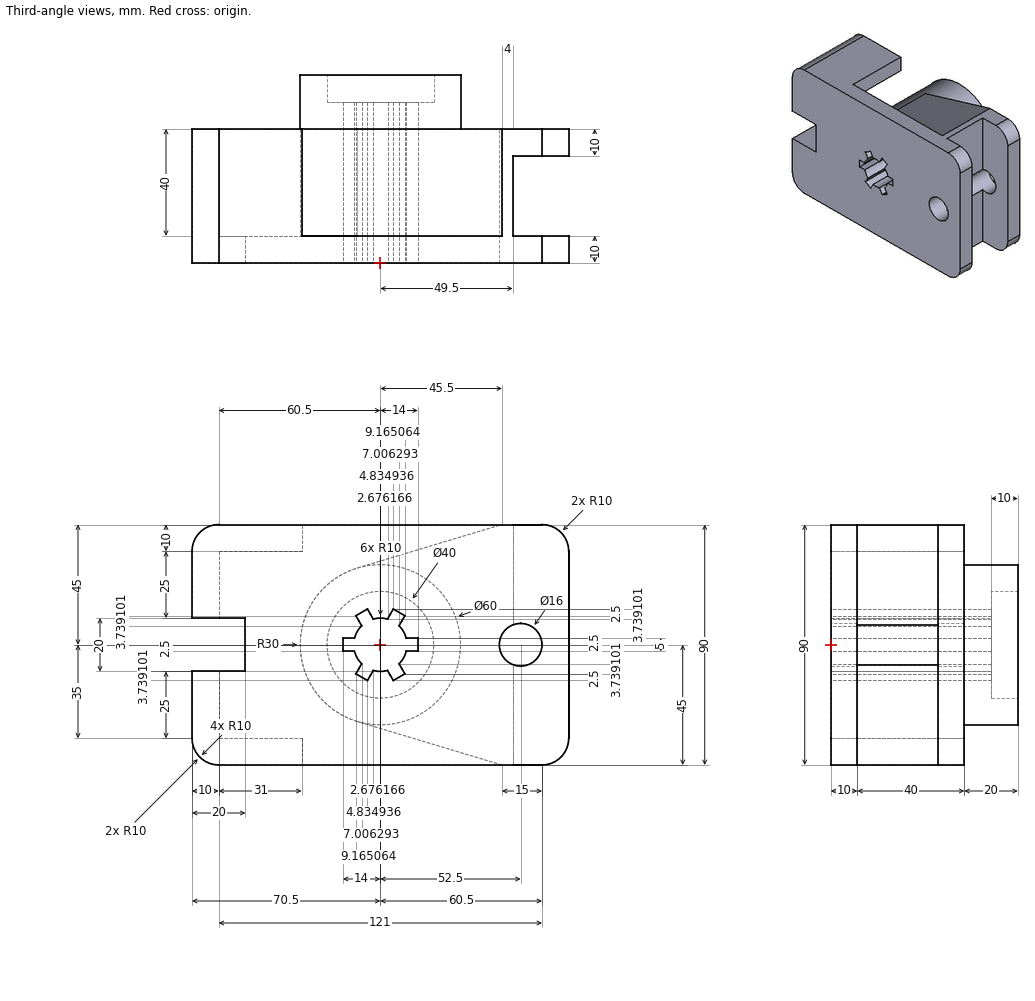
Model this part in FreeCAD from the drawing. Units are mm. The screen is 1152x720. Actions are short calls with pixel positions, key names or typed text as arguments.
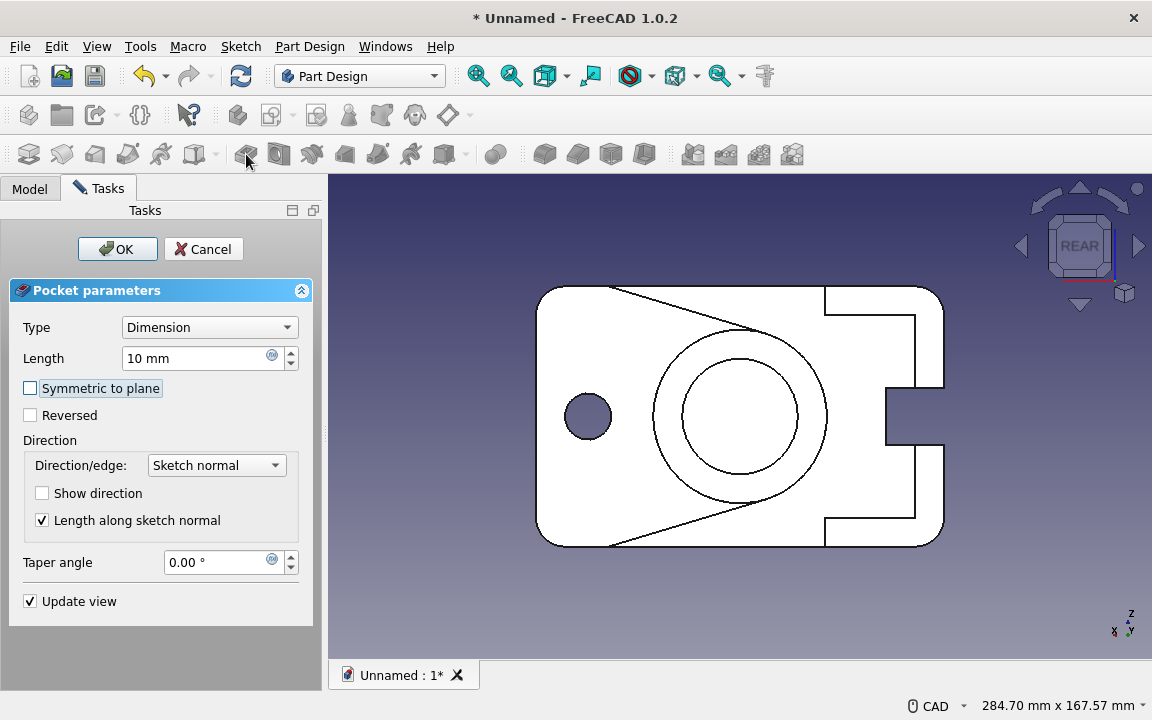
click(118, 249)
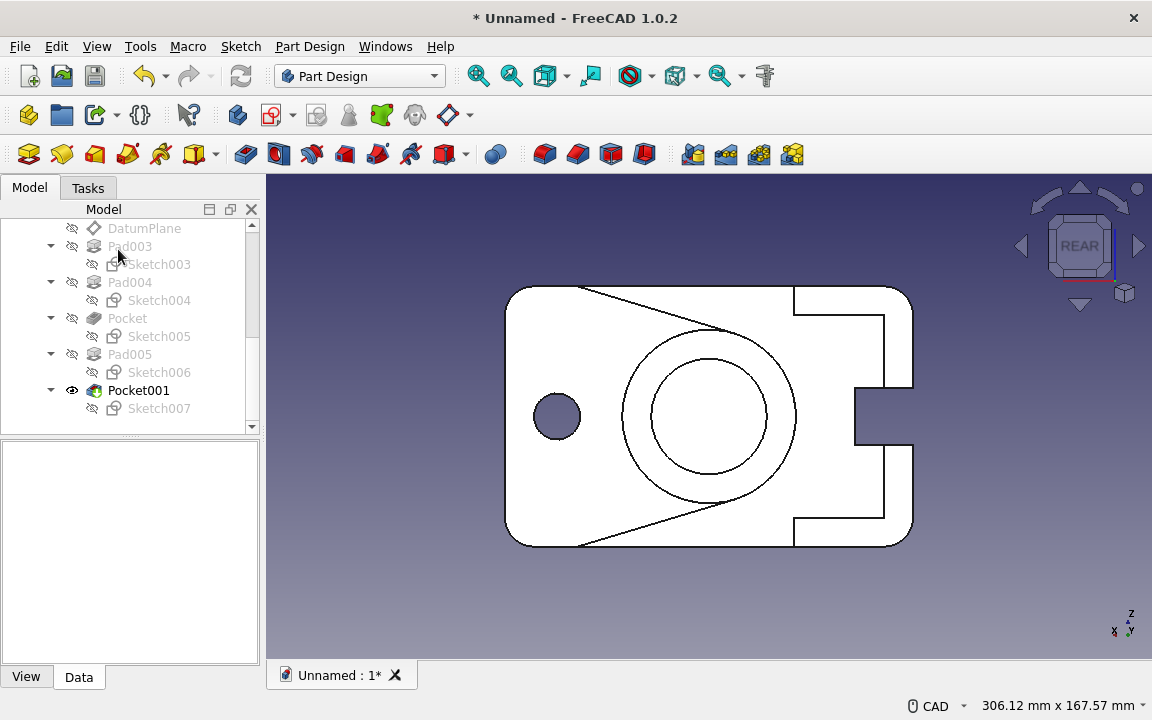
click(709, 416)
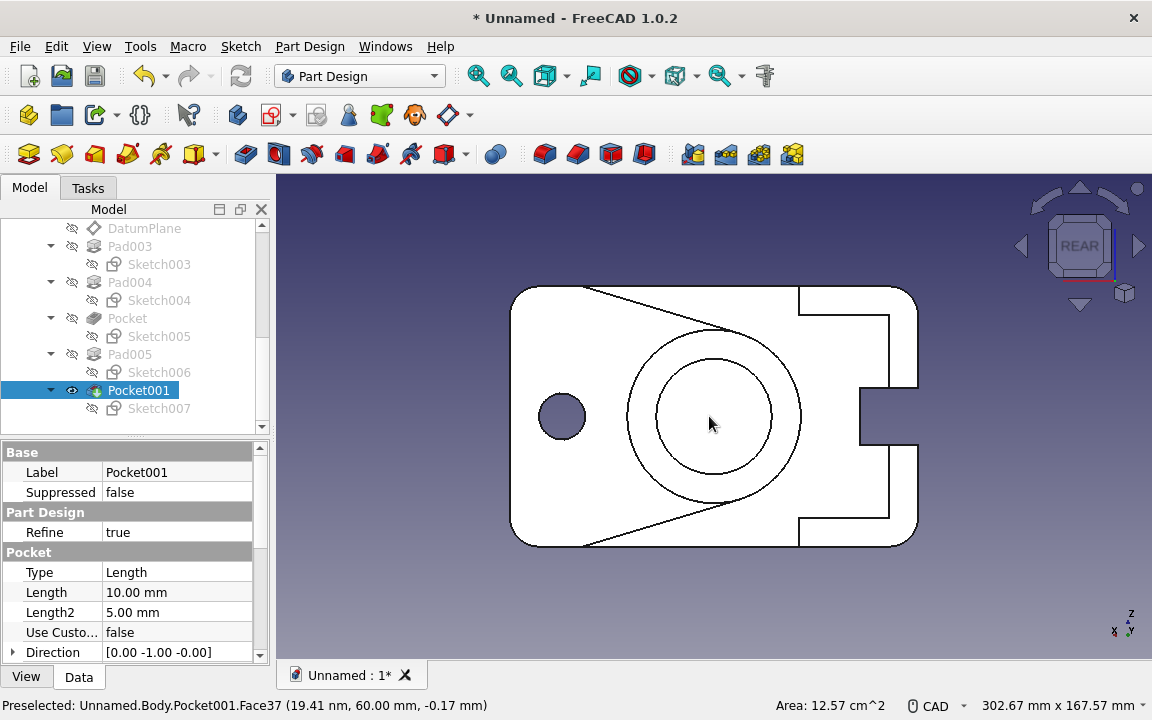
click(270, 116)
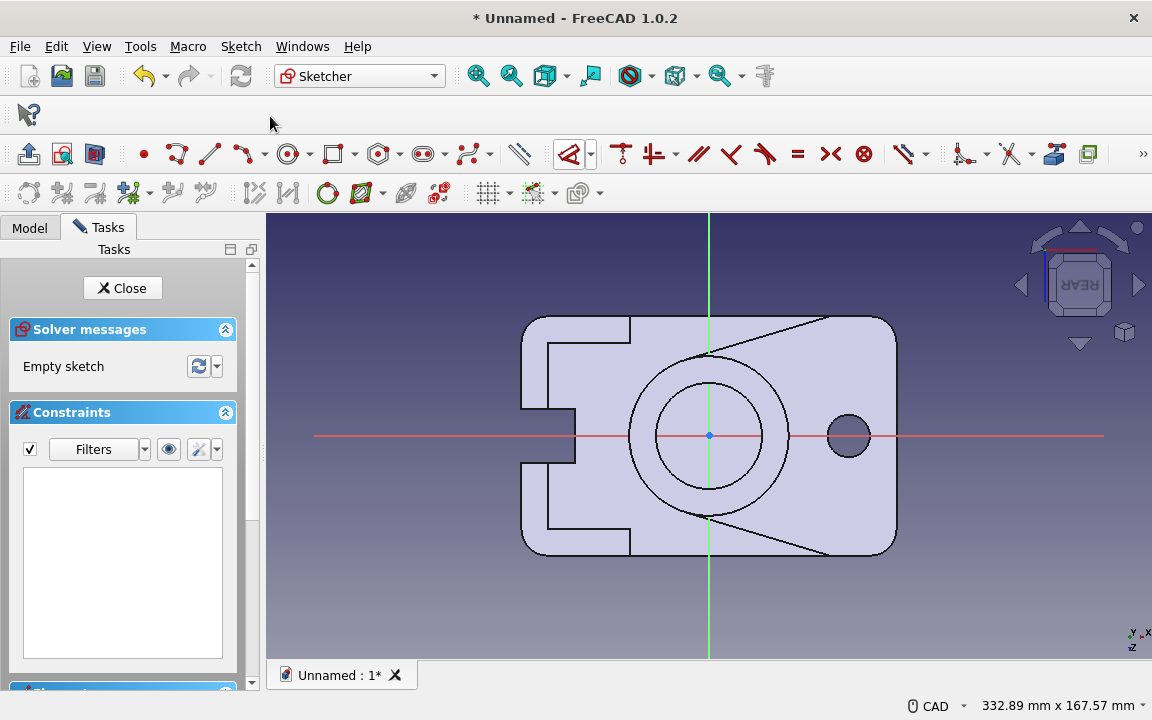
click(95, 154)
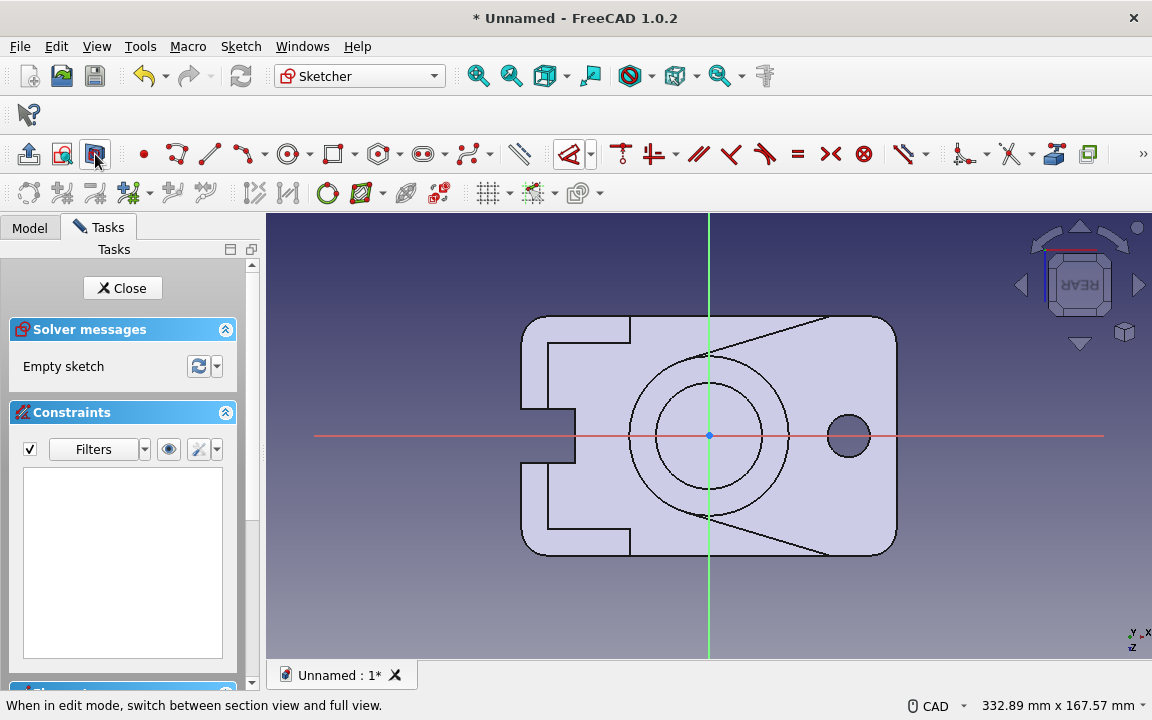
scroll(731, 436, up, 7)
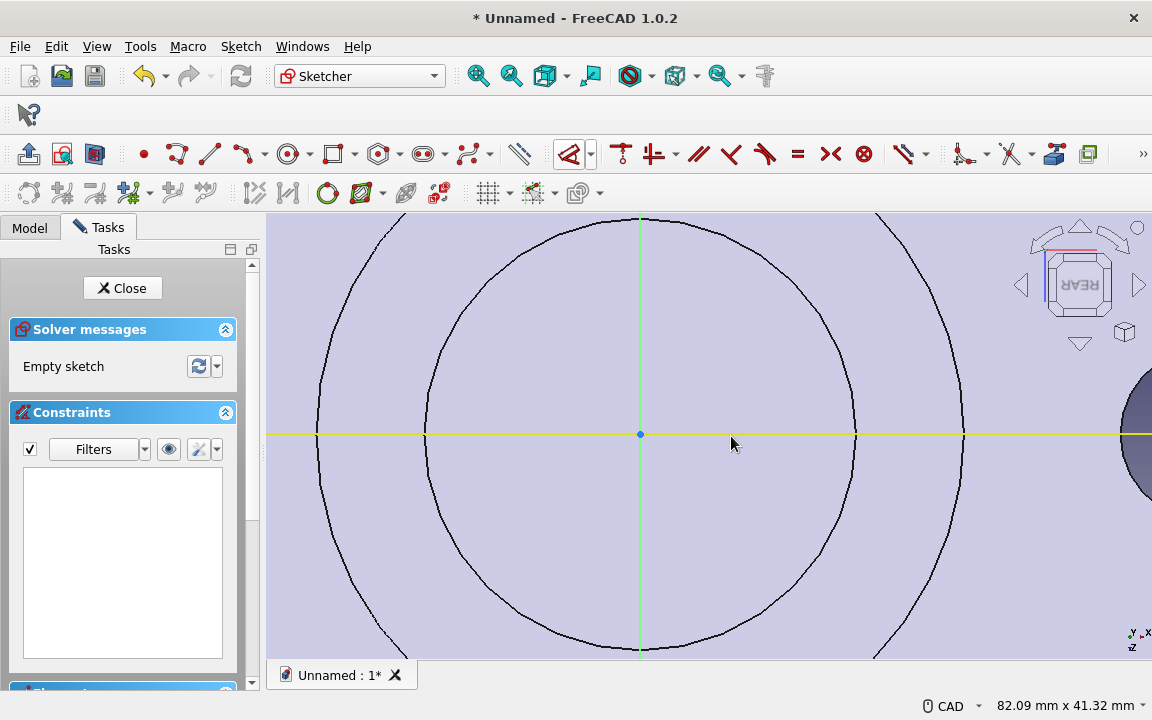
click(177, 154)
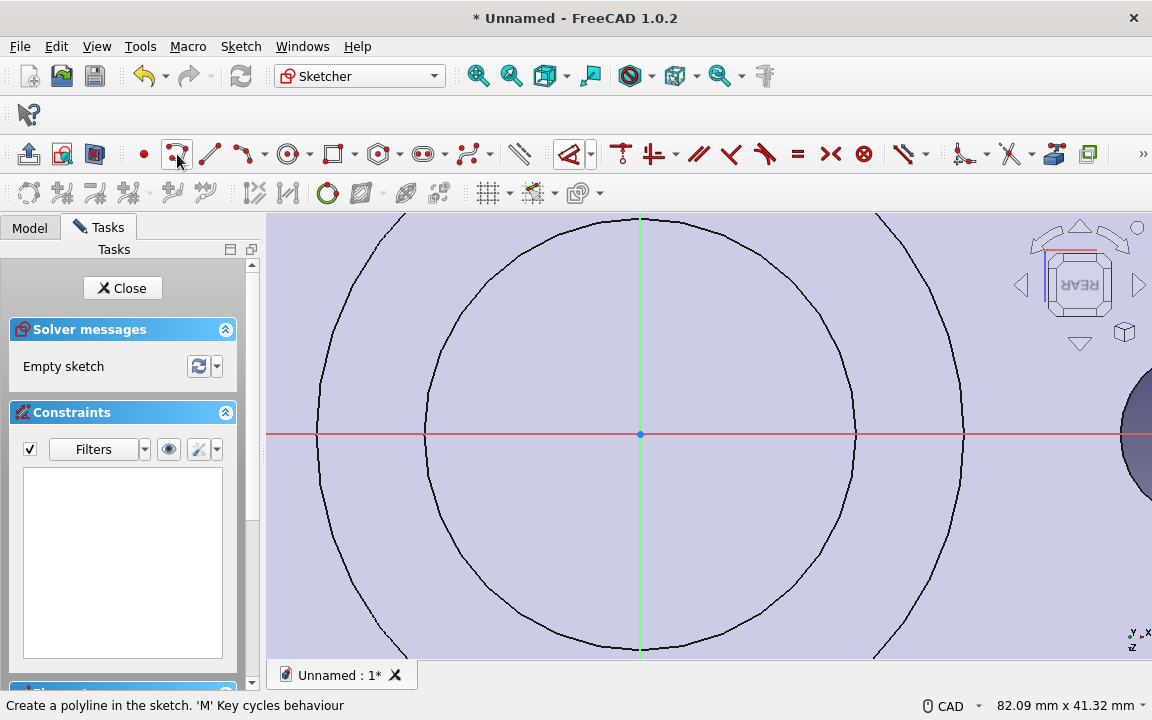
click(669, 538)
click(692, 579)
click(739, 552)
click(716, 511)
right_click(716, 511)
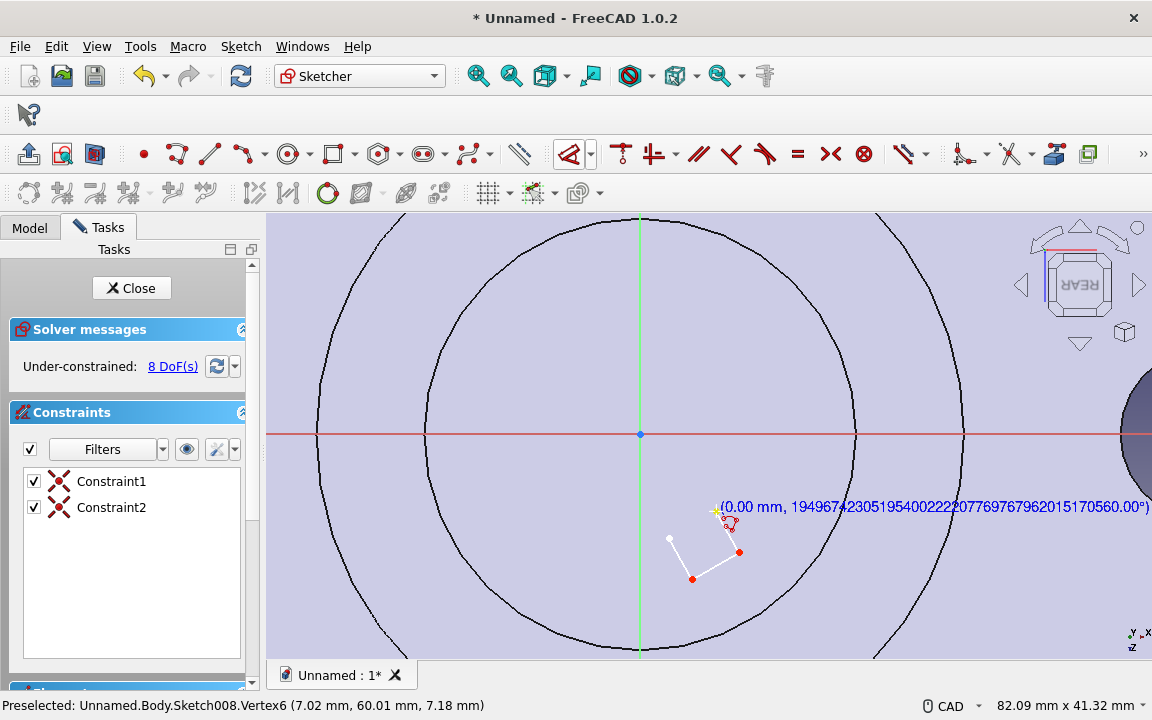
click(745, 461)
click(791, 461)
click(791, 407)
click(745, 407)
right_click(745, 407)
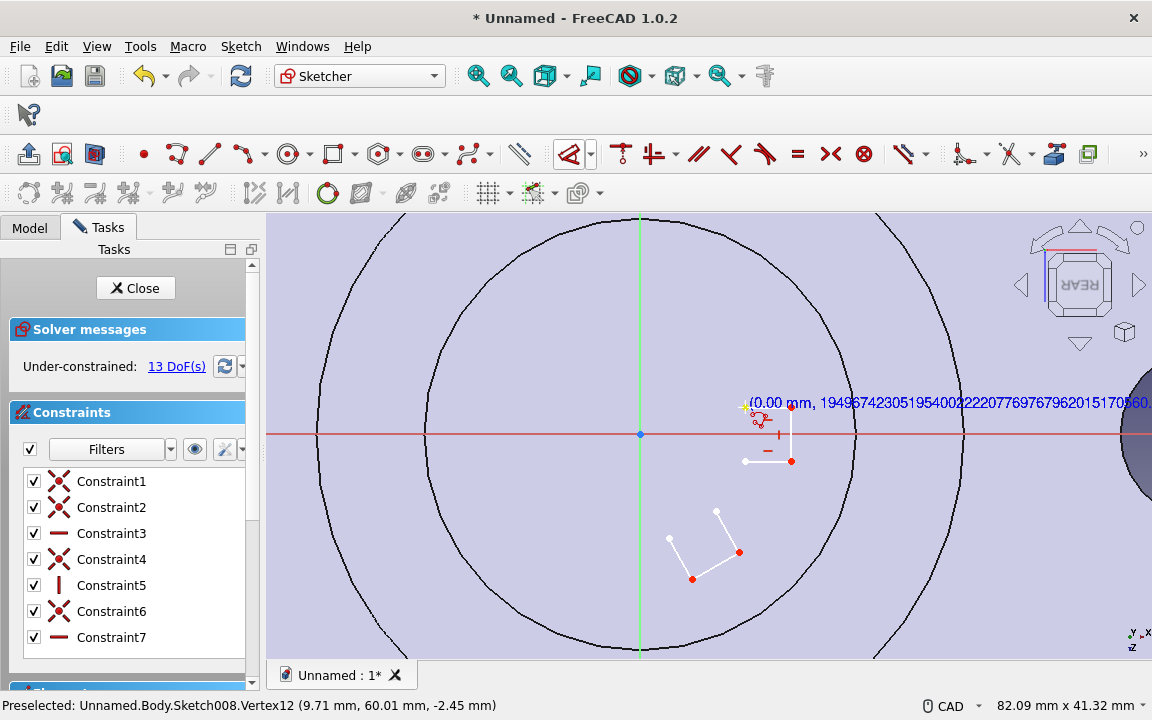
click(716, 357)
click(739, 317)
click(692, 290)
click(669, 330)
right_click(669, 330)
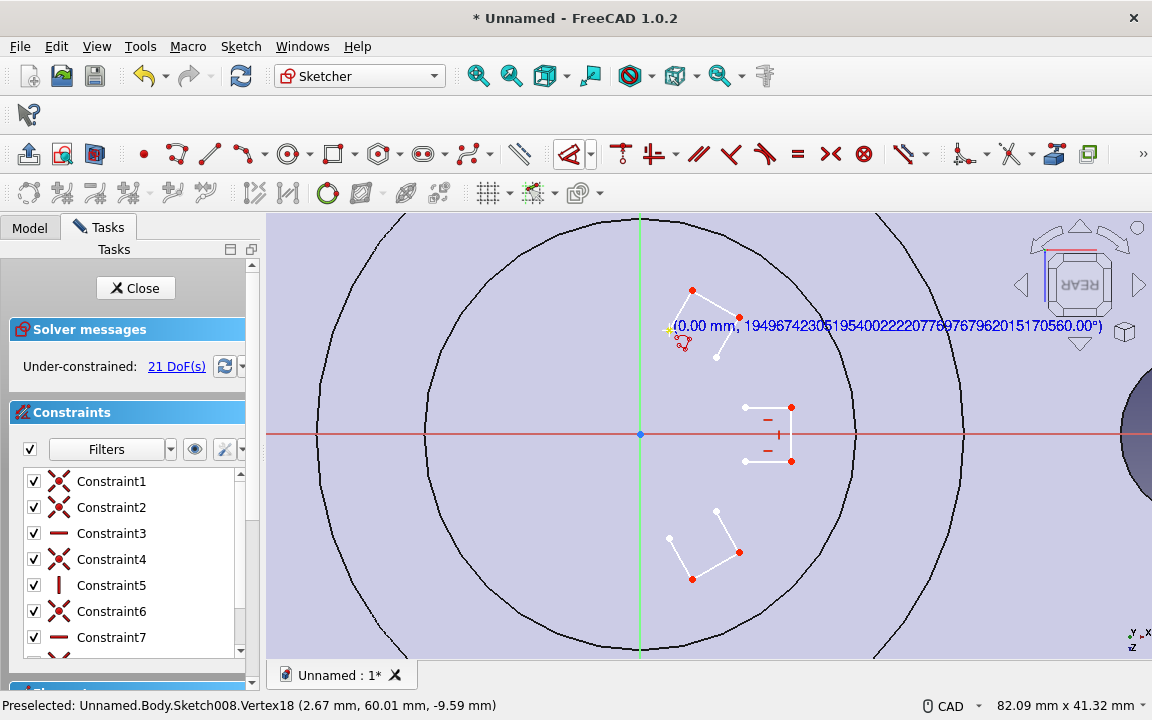
click(611, 330)
click(588, 290)
click(541, 317)
click(565, 357)
right_click(565, 357)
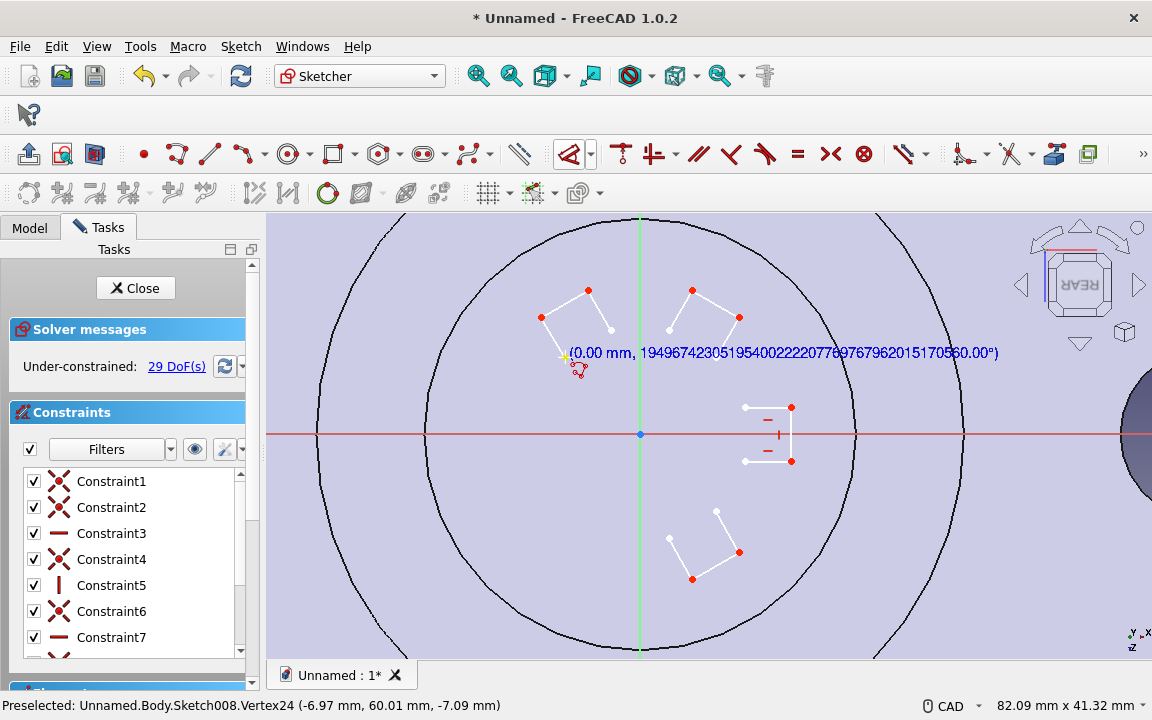
click(536, 407)
click(489, 407)
click(489, 461)
click(536, 461)
right_click(536, 461)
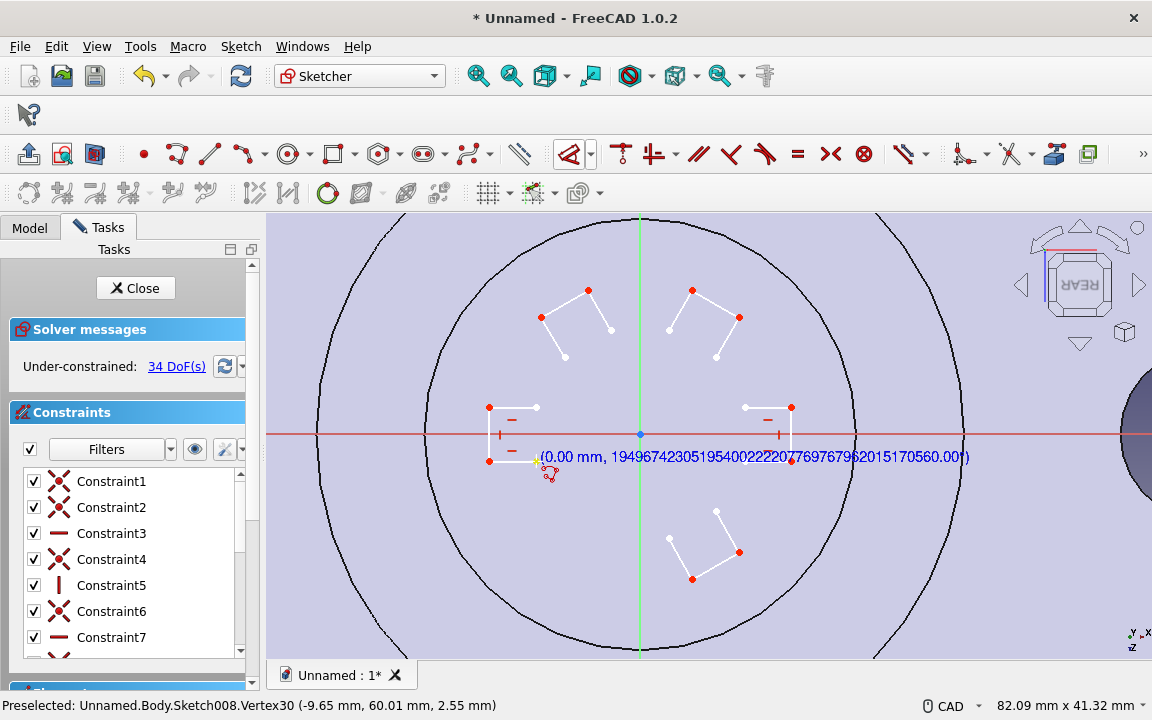
click(565, 511)
click(541, 552)
click(588, 579)
click(611, 538)
right_click(611, 538)